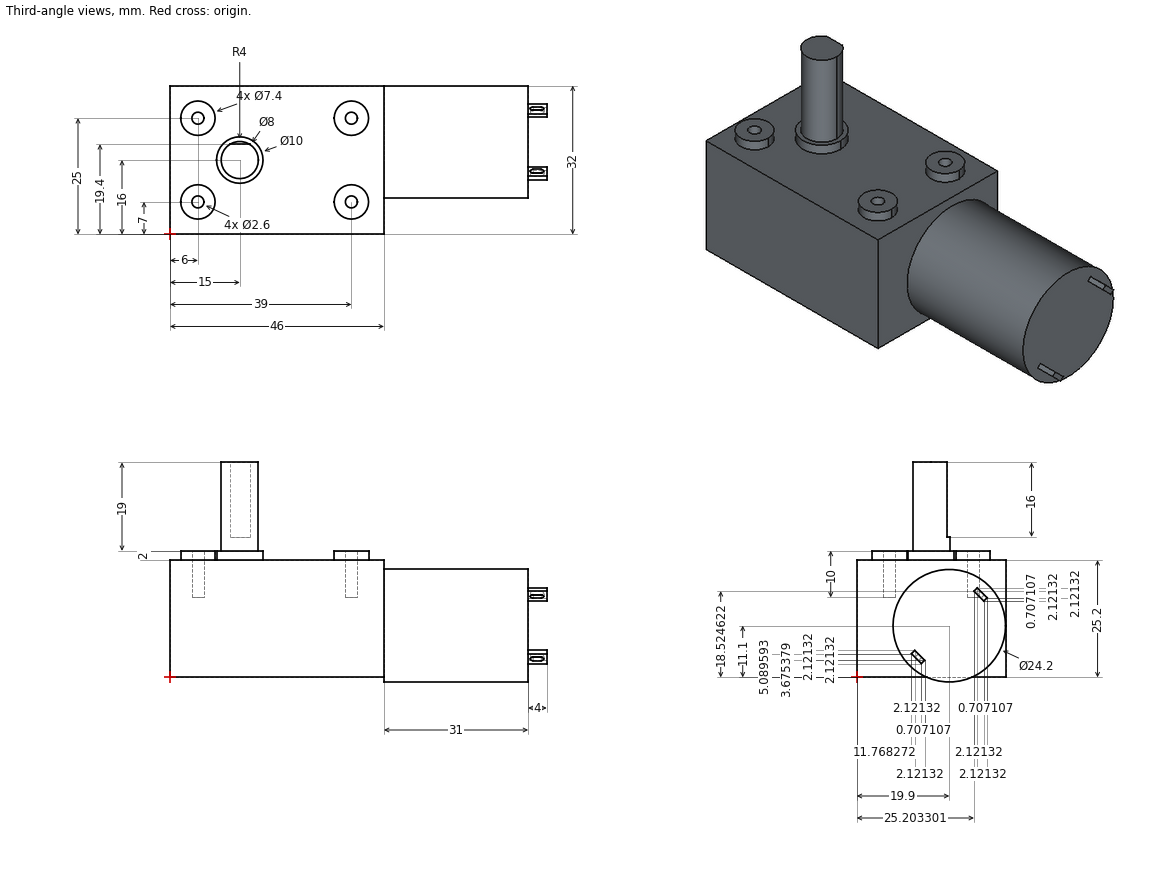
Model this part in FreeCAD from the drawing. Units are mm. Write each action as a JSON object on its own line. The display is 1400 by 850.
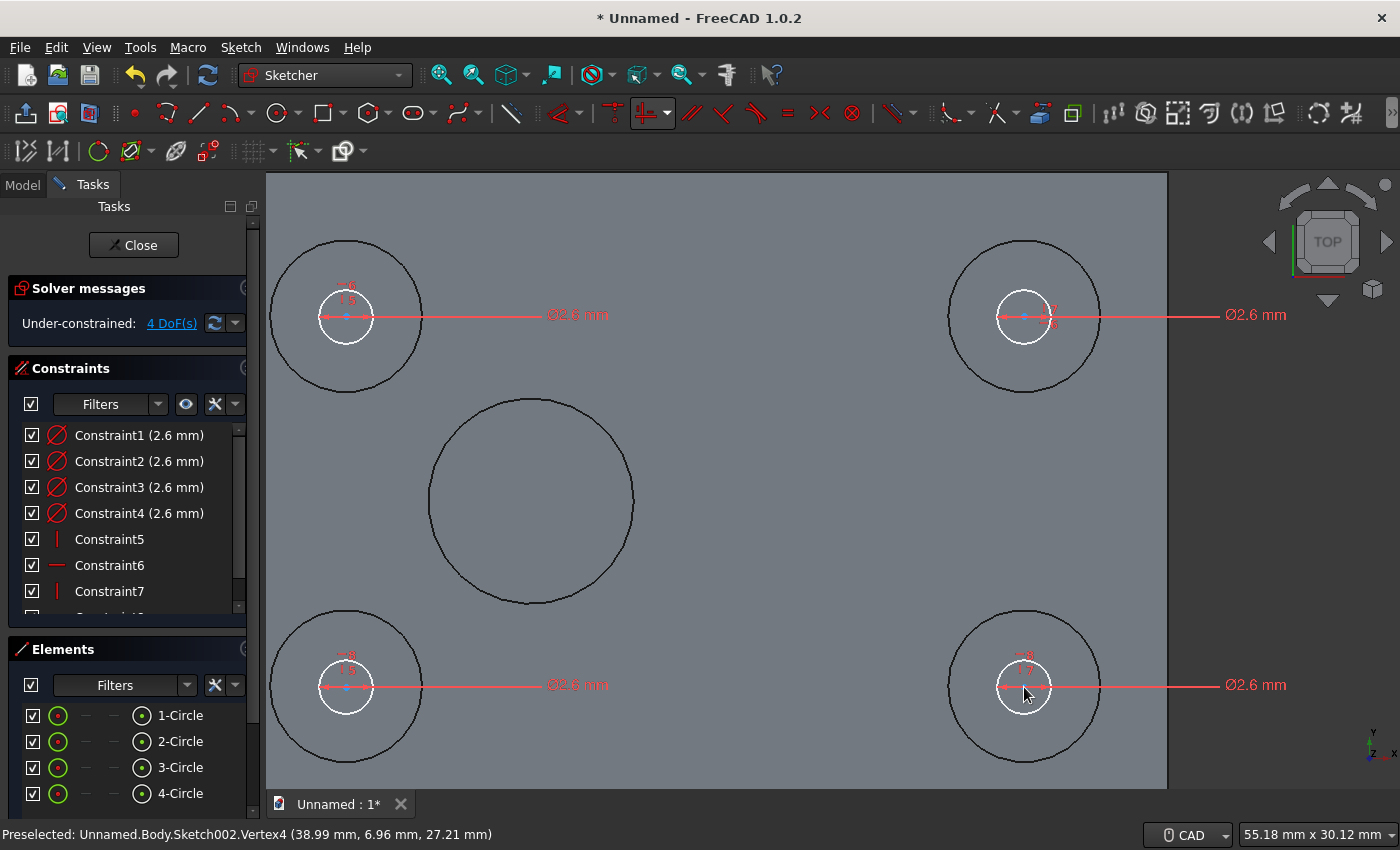
{"action": "left_click", "coordinate": [558, 114]}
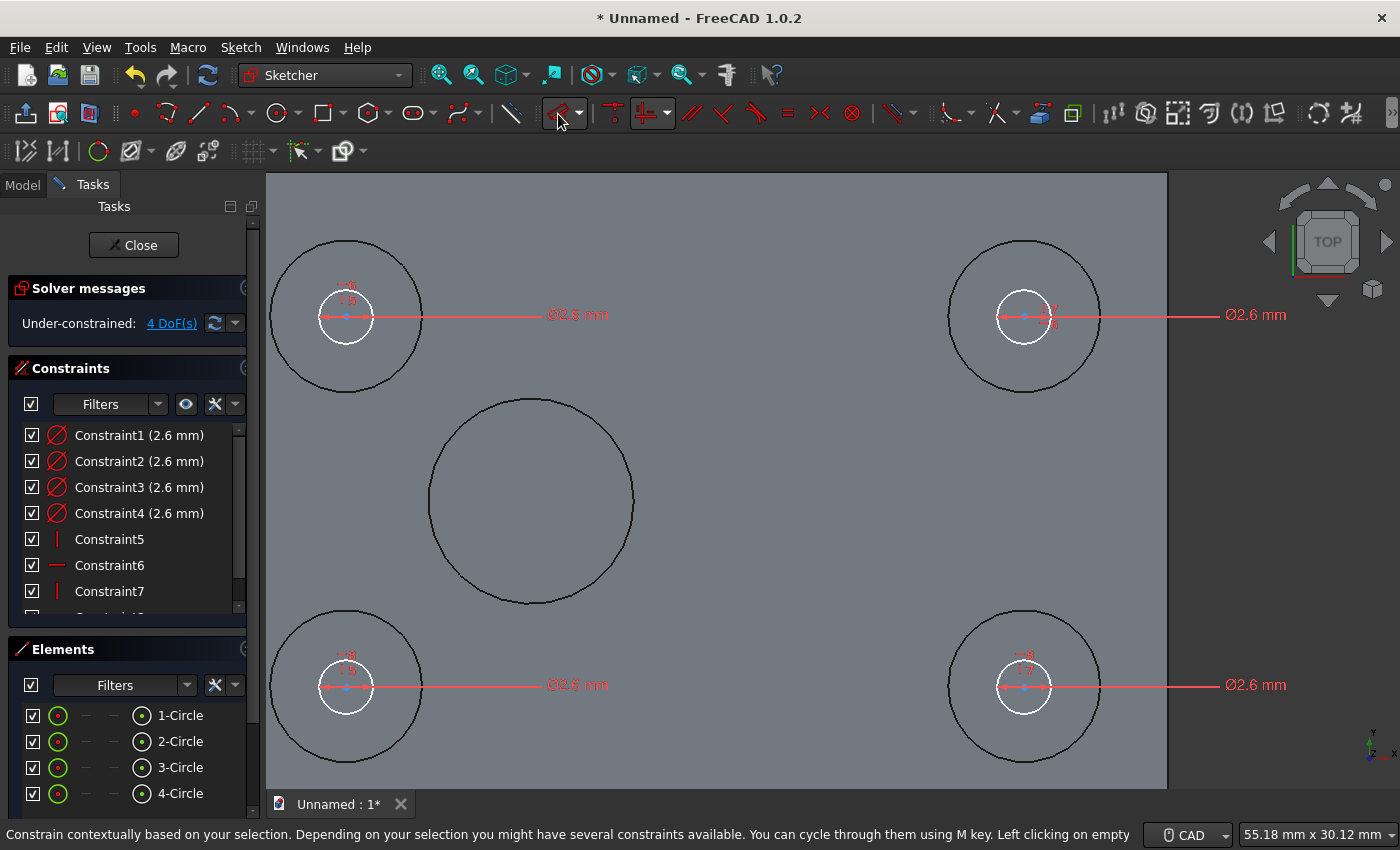
{"action": "left_click", "coordinate": [346, 687]}
{"action": "left_click", "coordinate": [320, 653]}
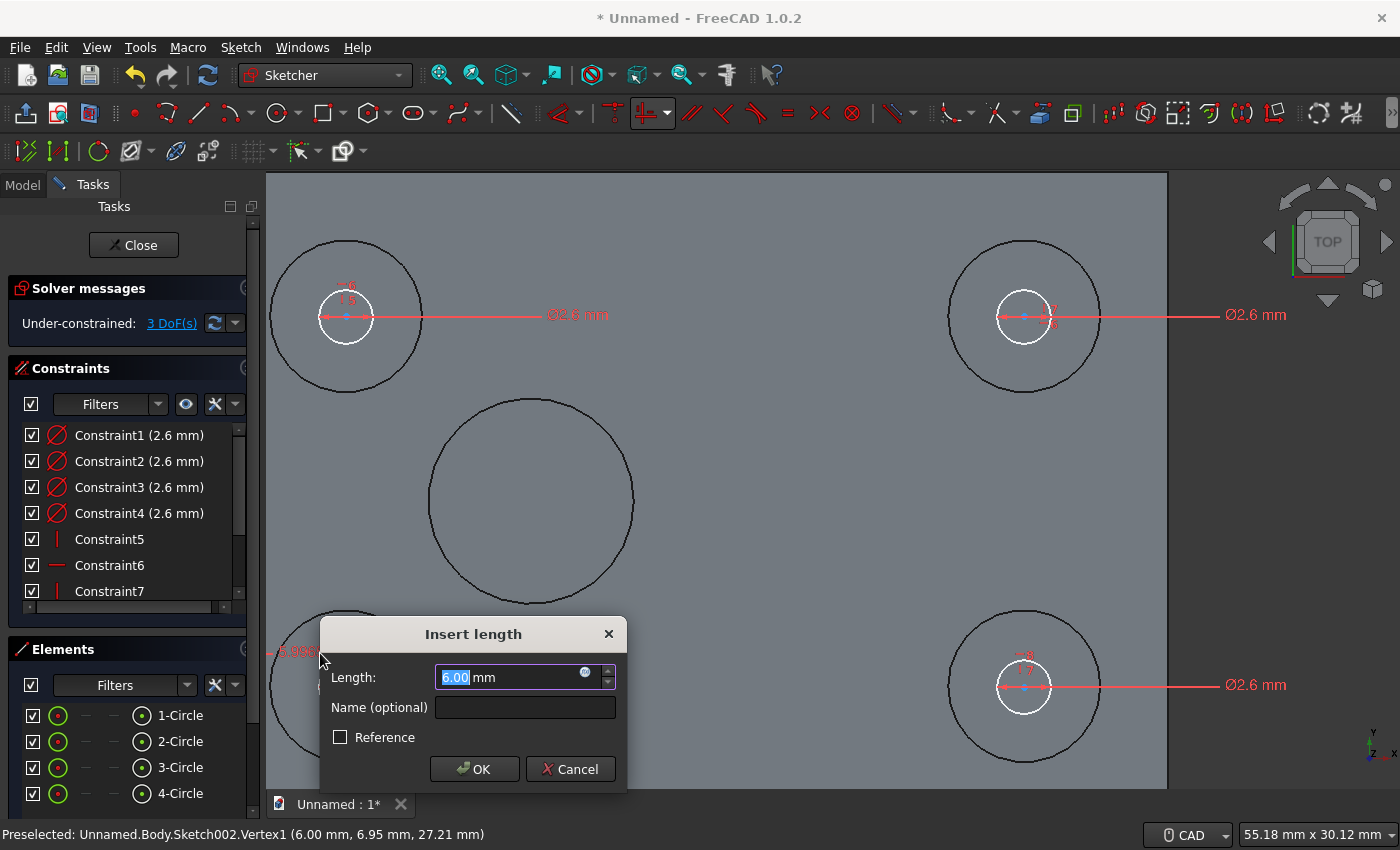
{"action": "type", "text": "6"}
{"action": "key", "text": "Return"}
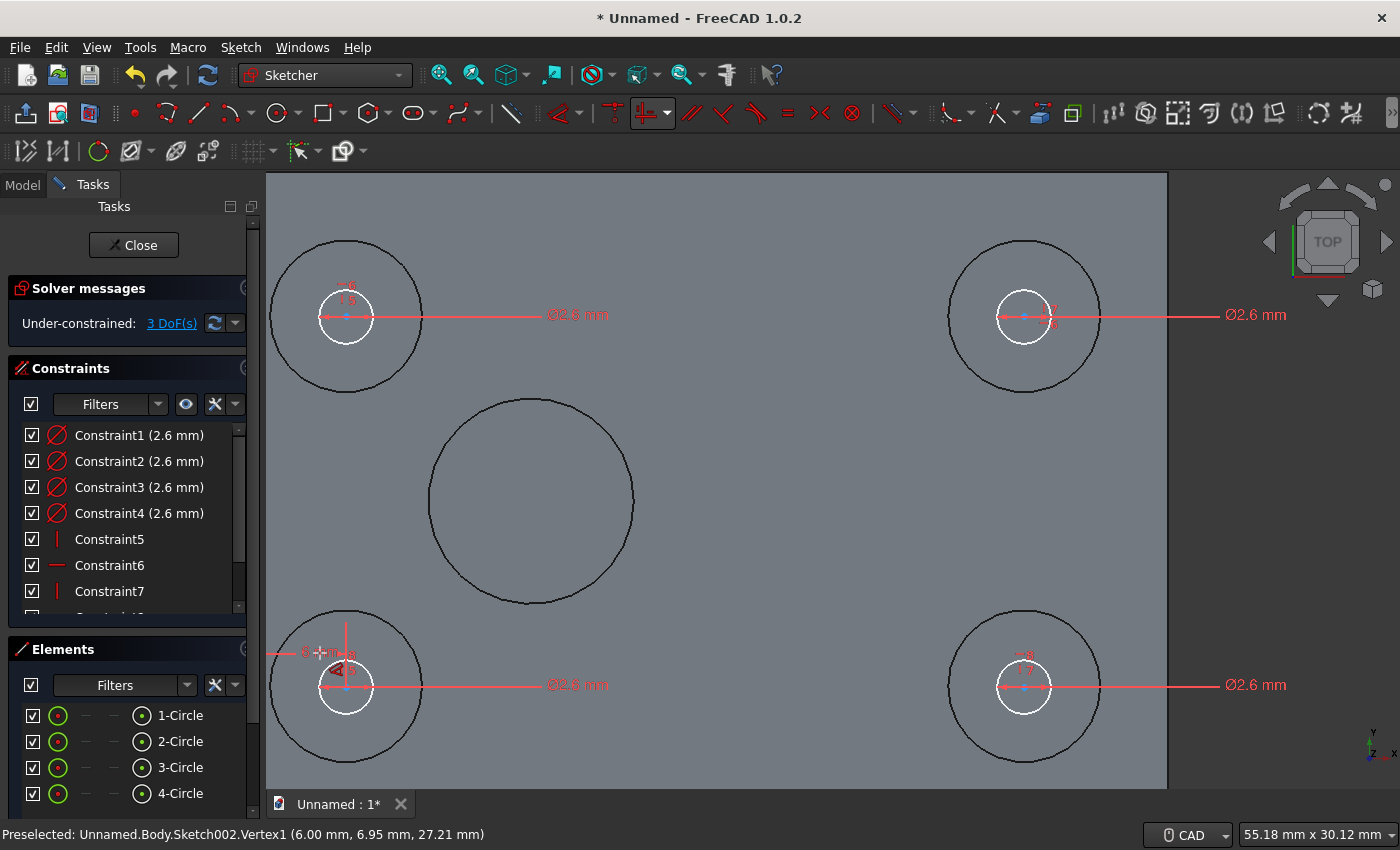
{"action": "left_click", "coordinate": [346, 687]}
{"action": "left_click", "coordinate": [380, 724]}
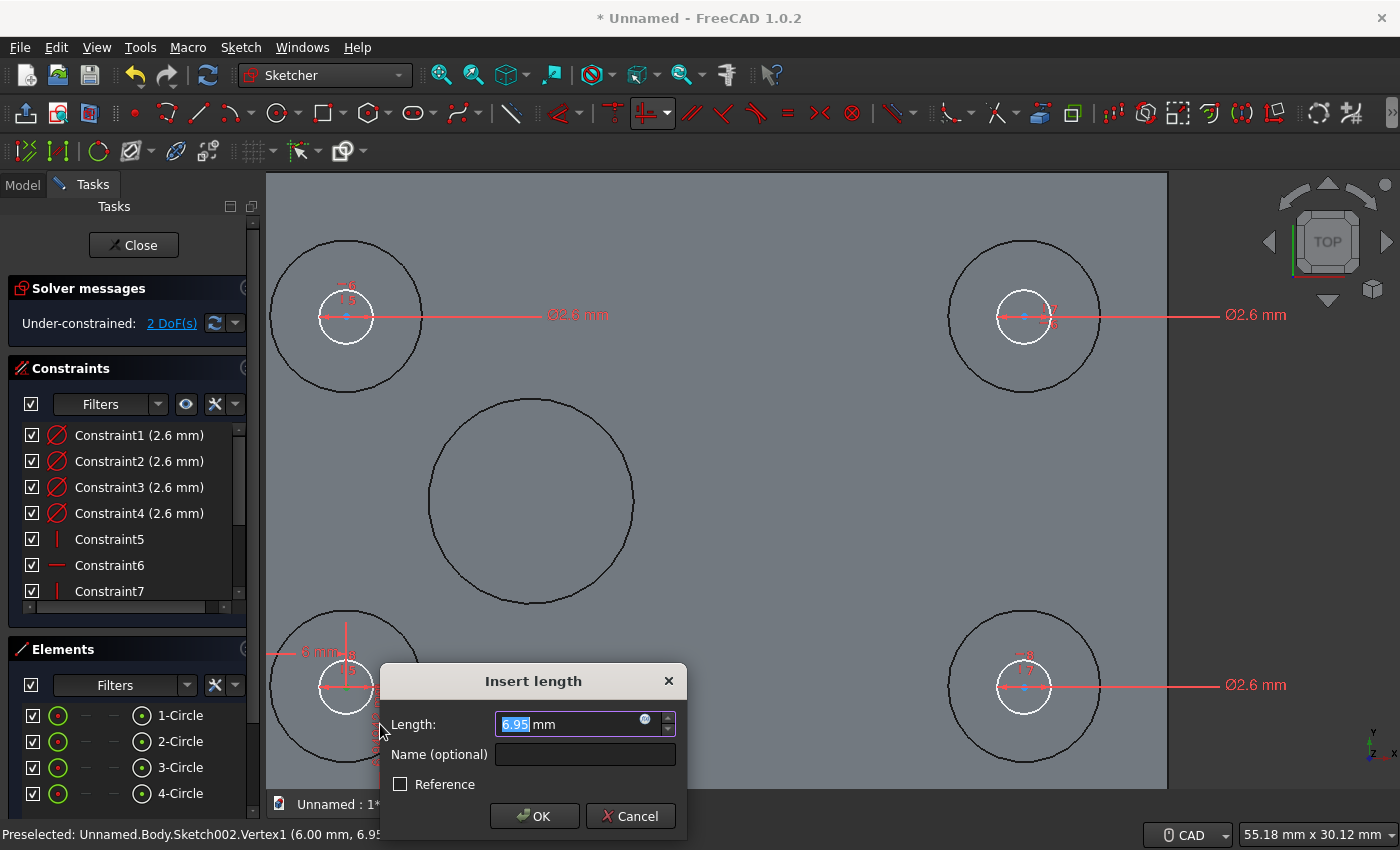
{"action": "type", "text": "7"}
{"action": "key", "text": "Return"}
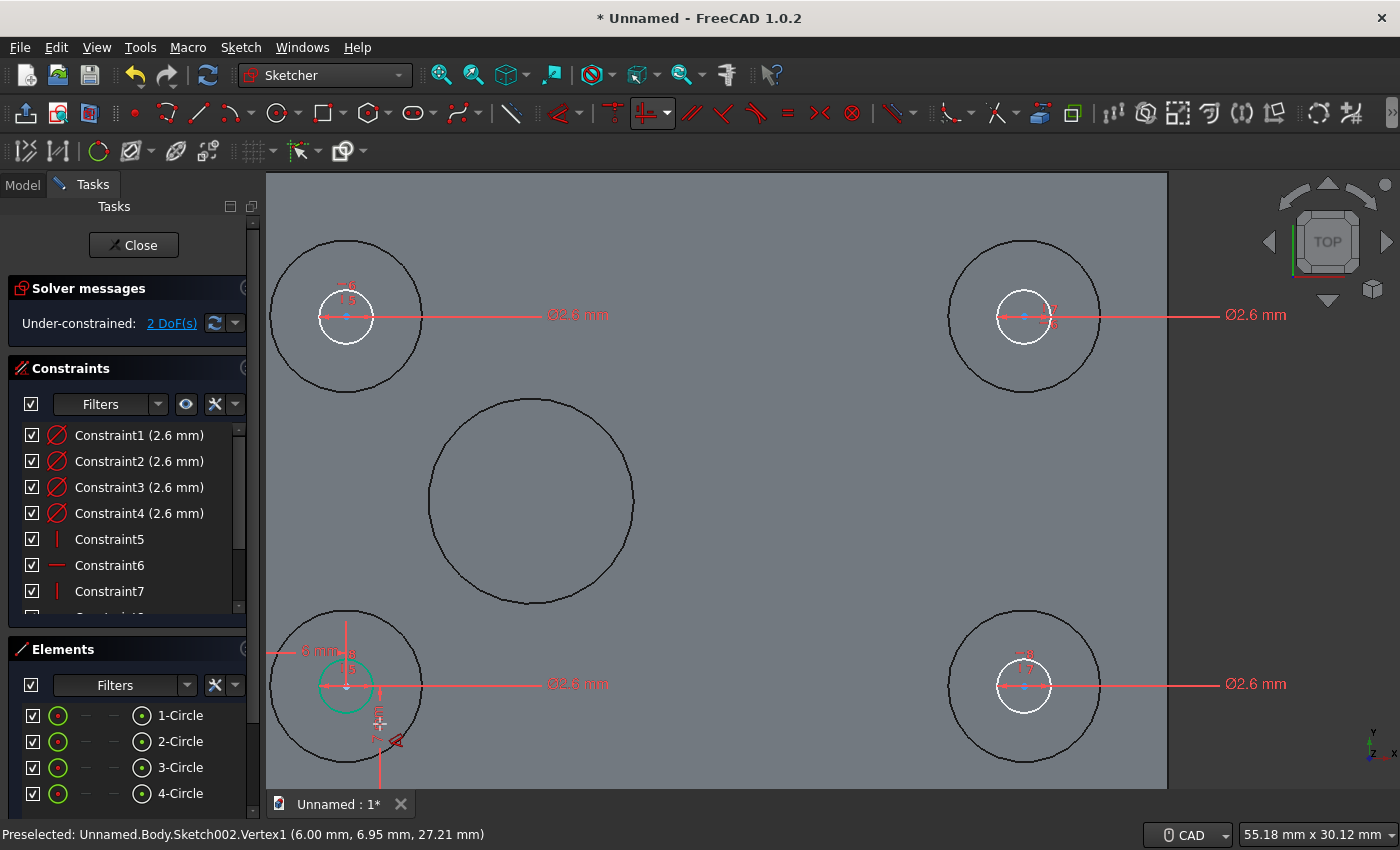
{"action": "left_click", "coordinate": [346, 317]}
{"action": "left_click", "coordinate": [380, 539]}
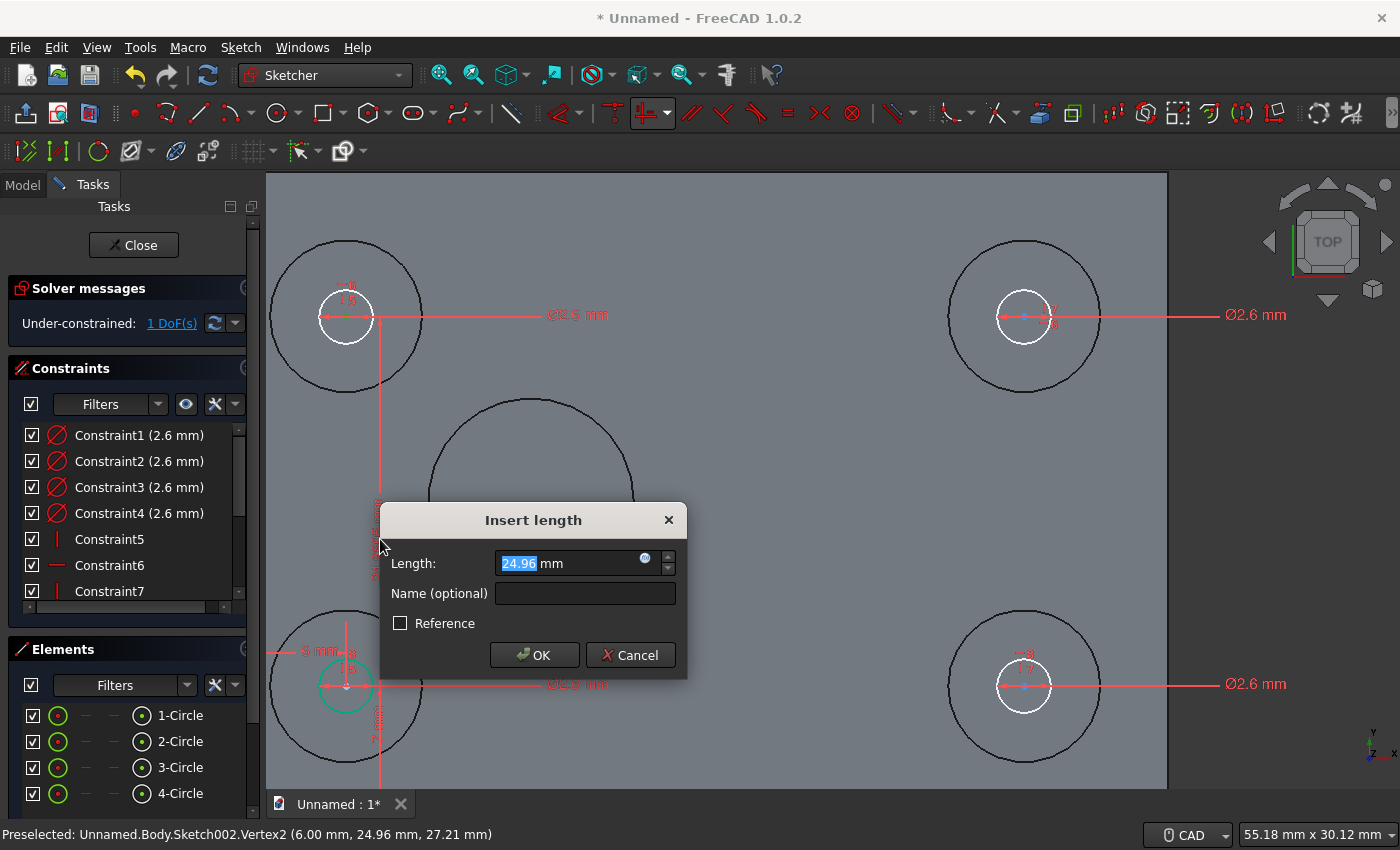
{"action": "type", "text": "25"}
{"action": "key", "text": "Return"}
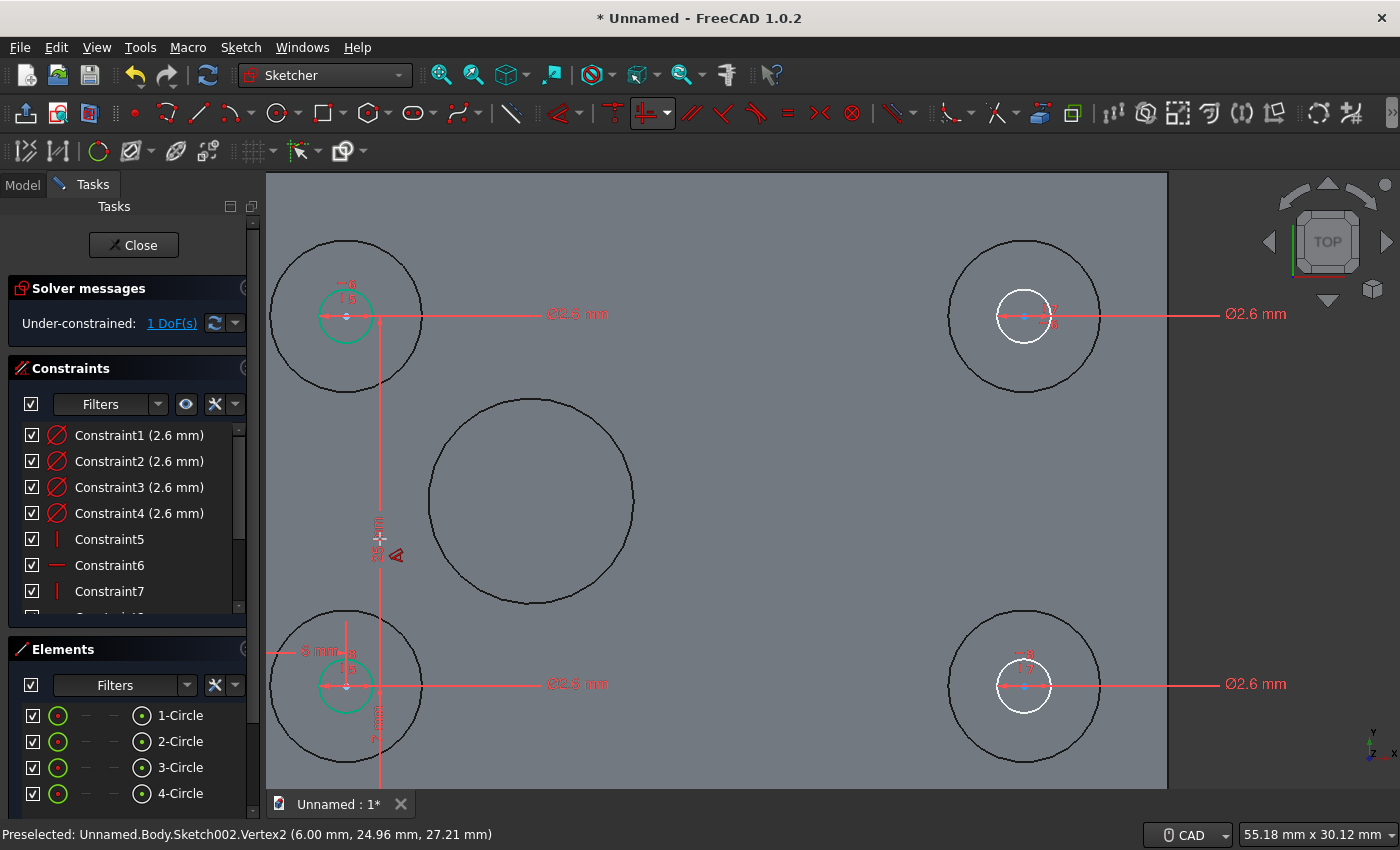
{"action": "left_click", "coordinate": [1024, 316]}
{"action": "left_click", "coordinate": [659, 282]}